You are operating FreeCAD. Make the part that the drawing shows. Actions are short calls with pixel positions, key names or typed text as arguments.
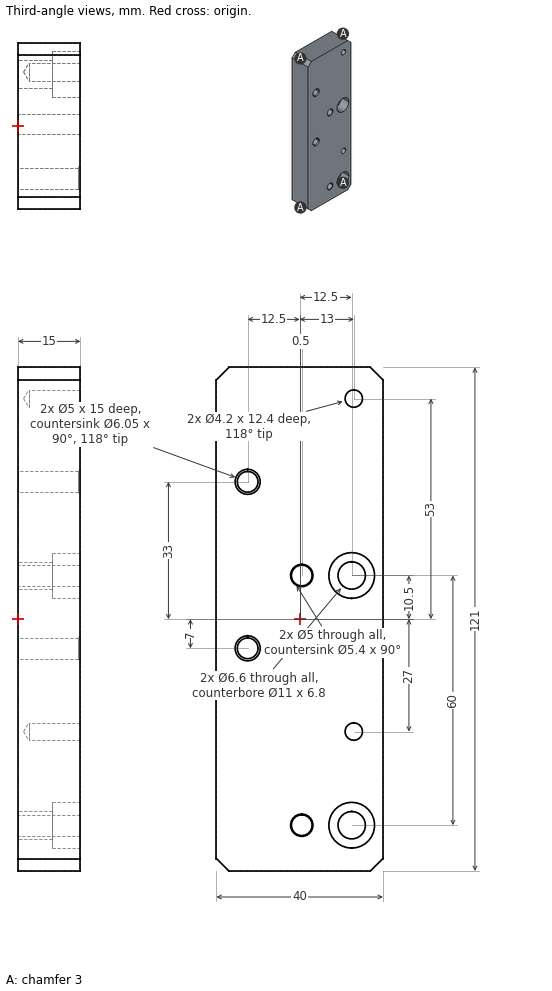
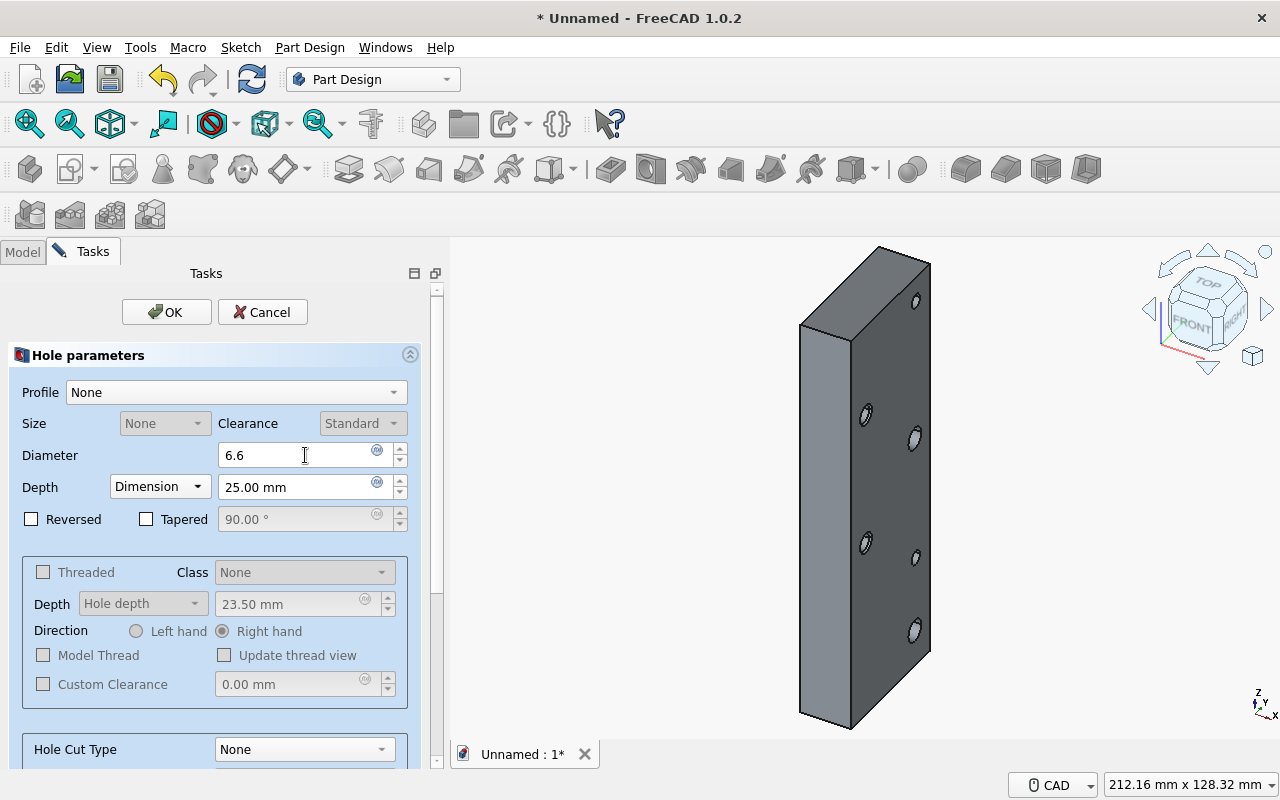
click(161, 486)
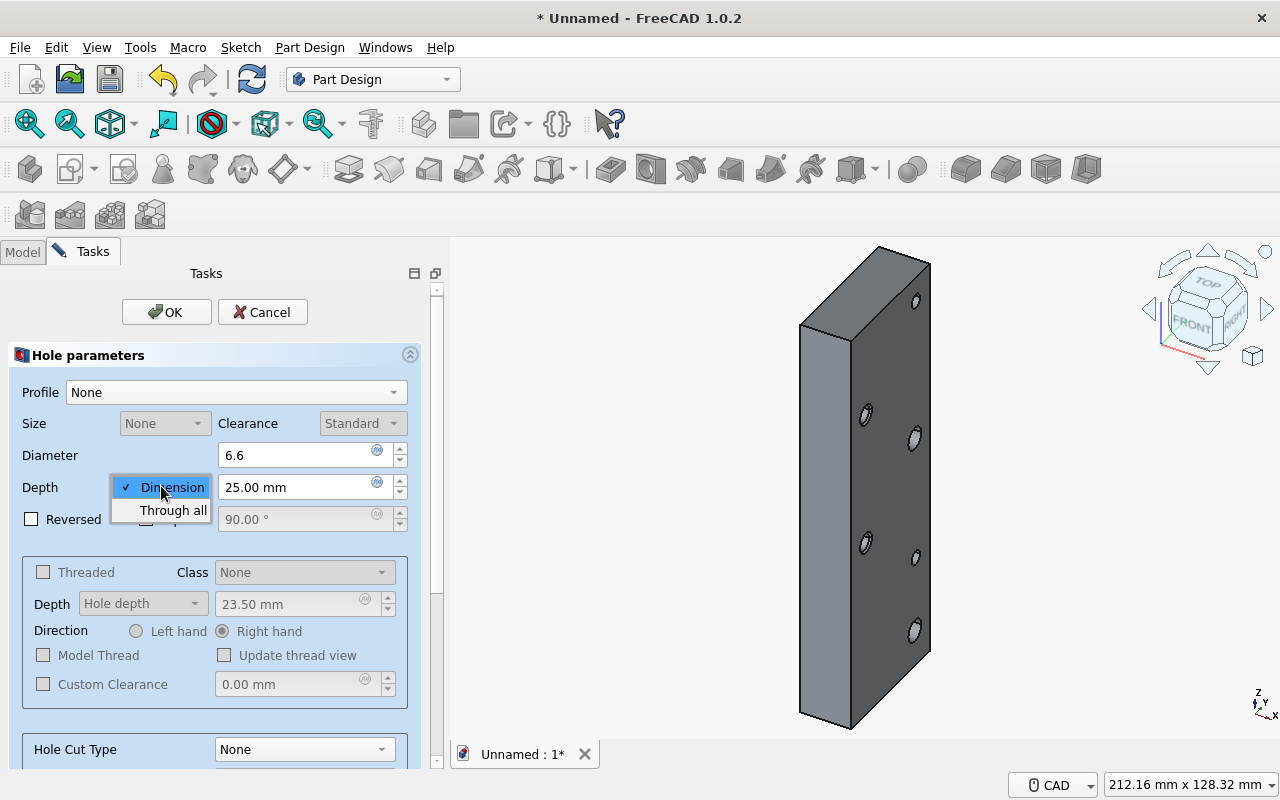
click(160, 510)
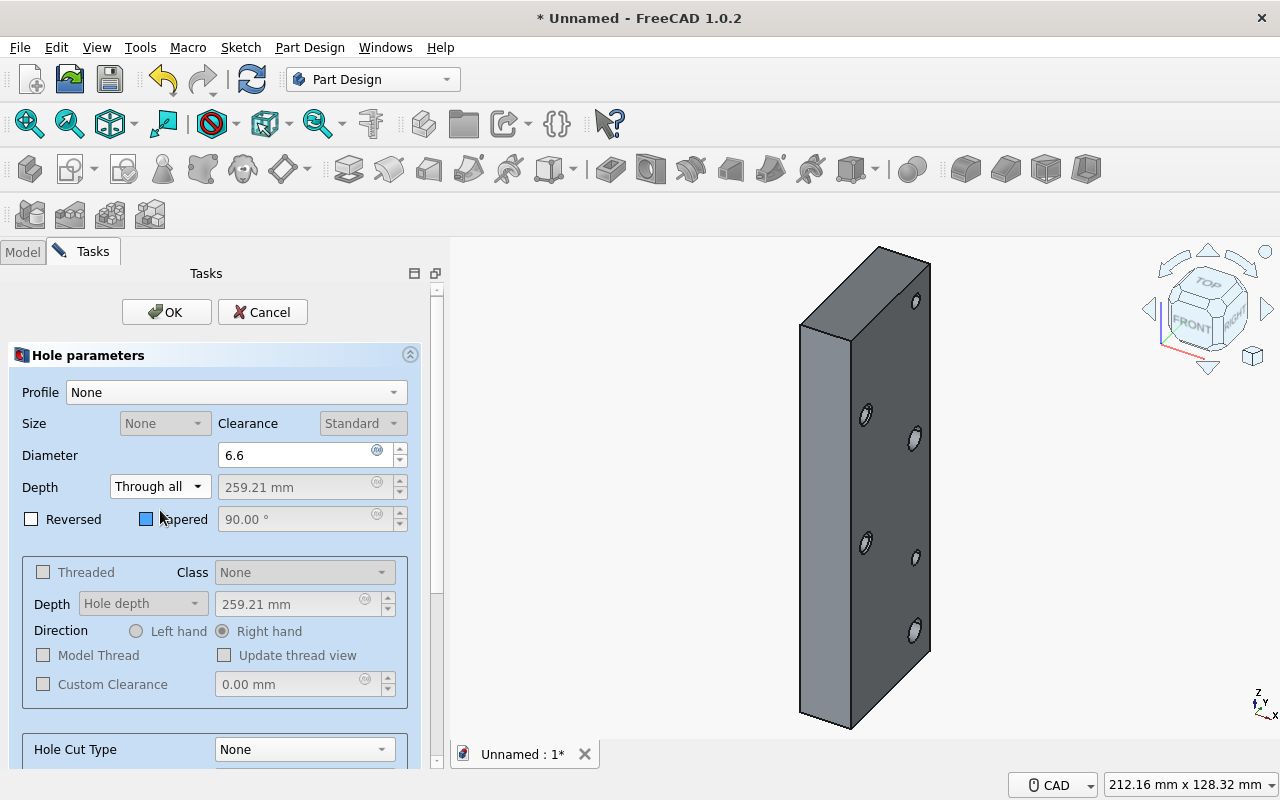
click(306, 750)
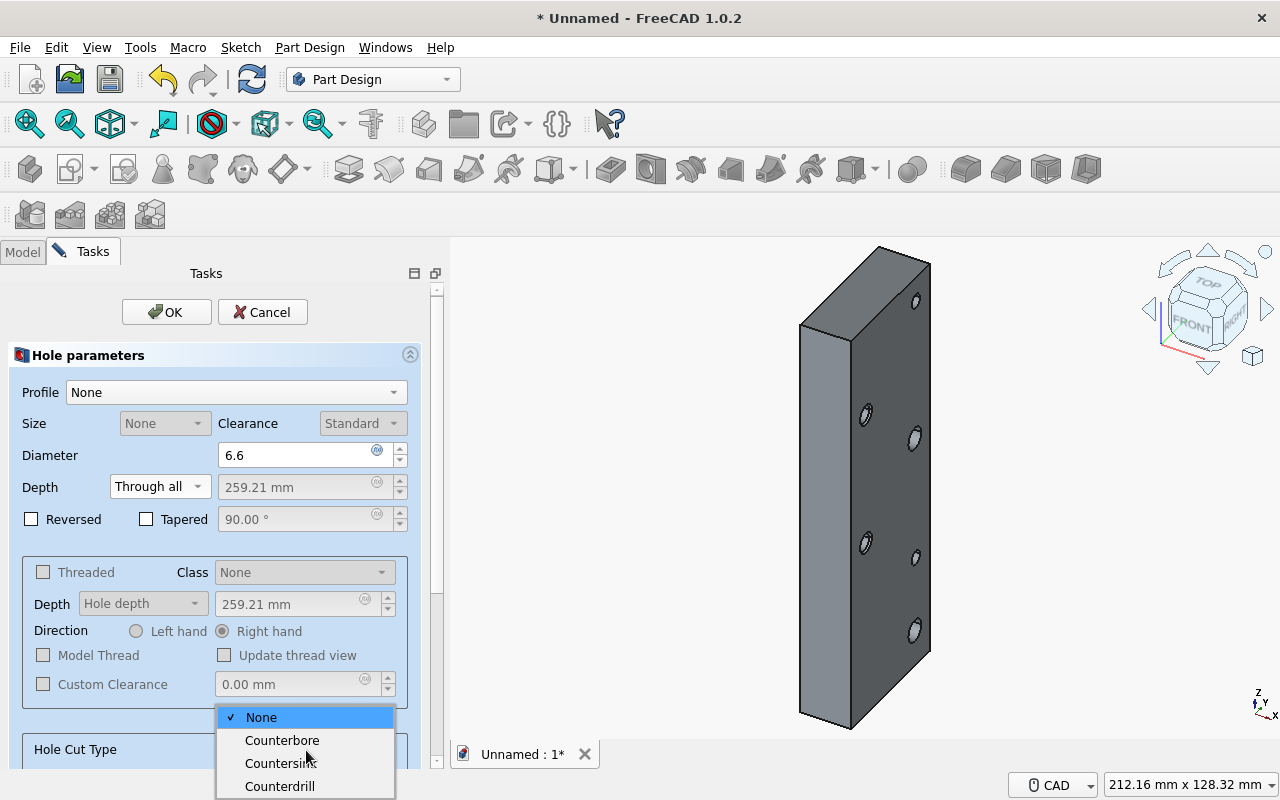
click(304, 740)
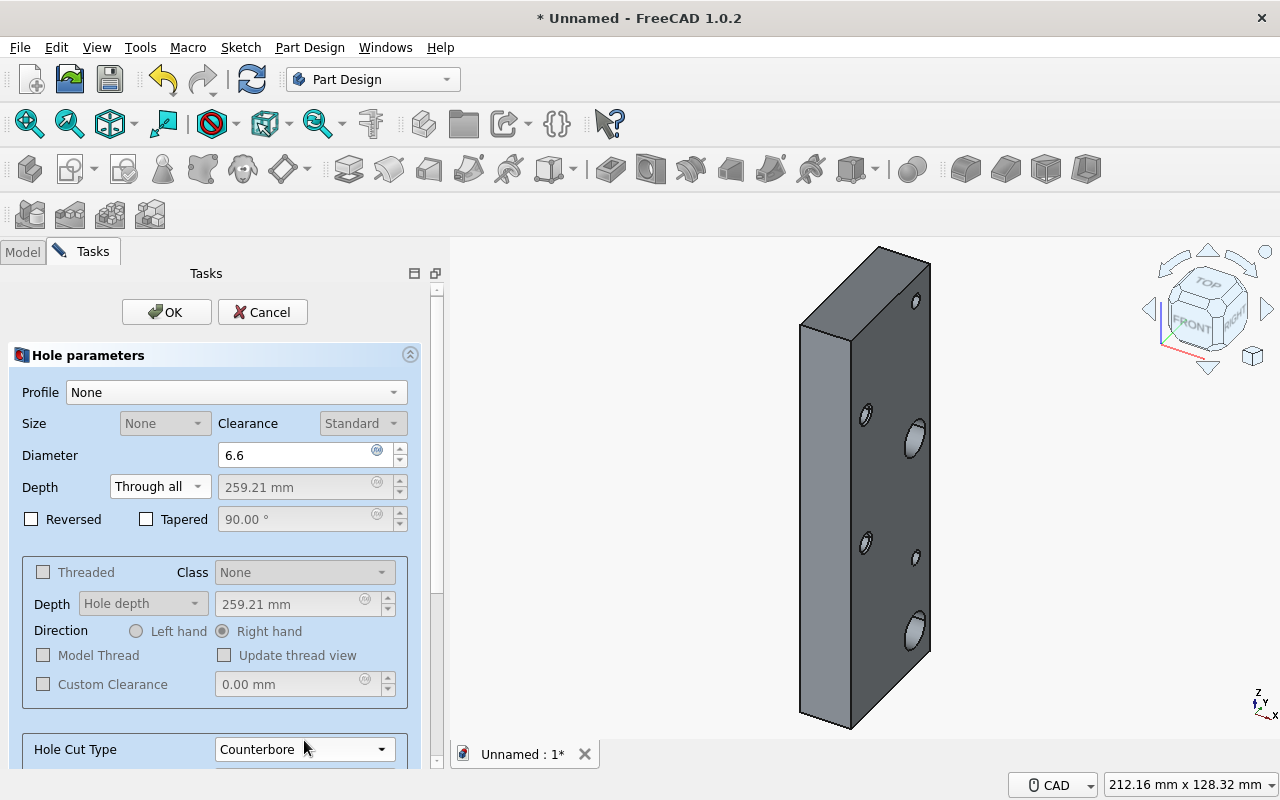
scroll(437, 526, down, 2)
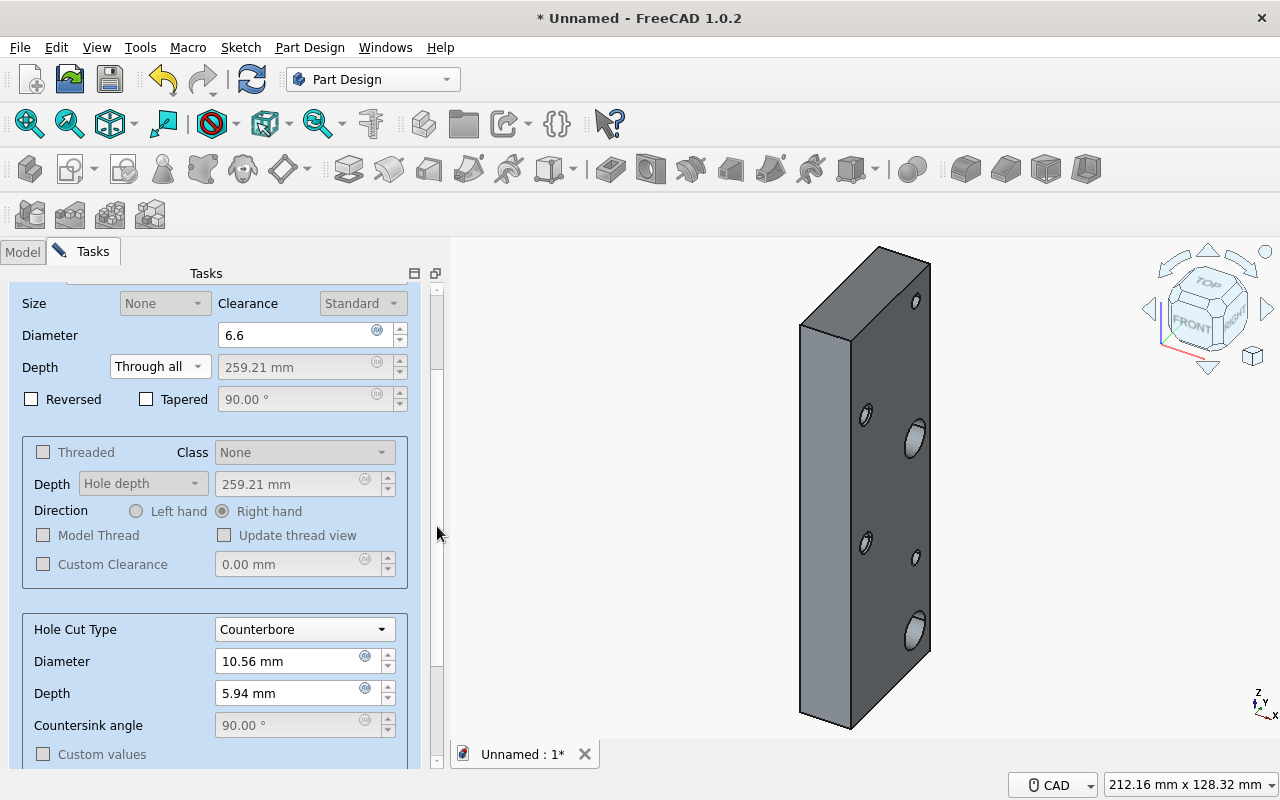
triple_click(298, 661)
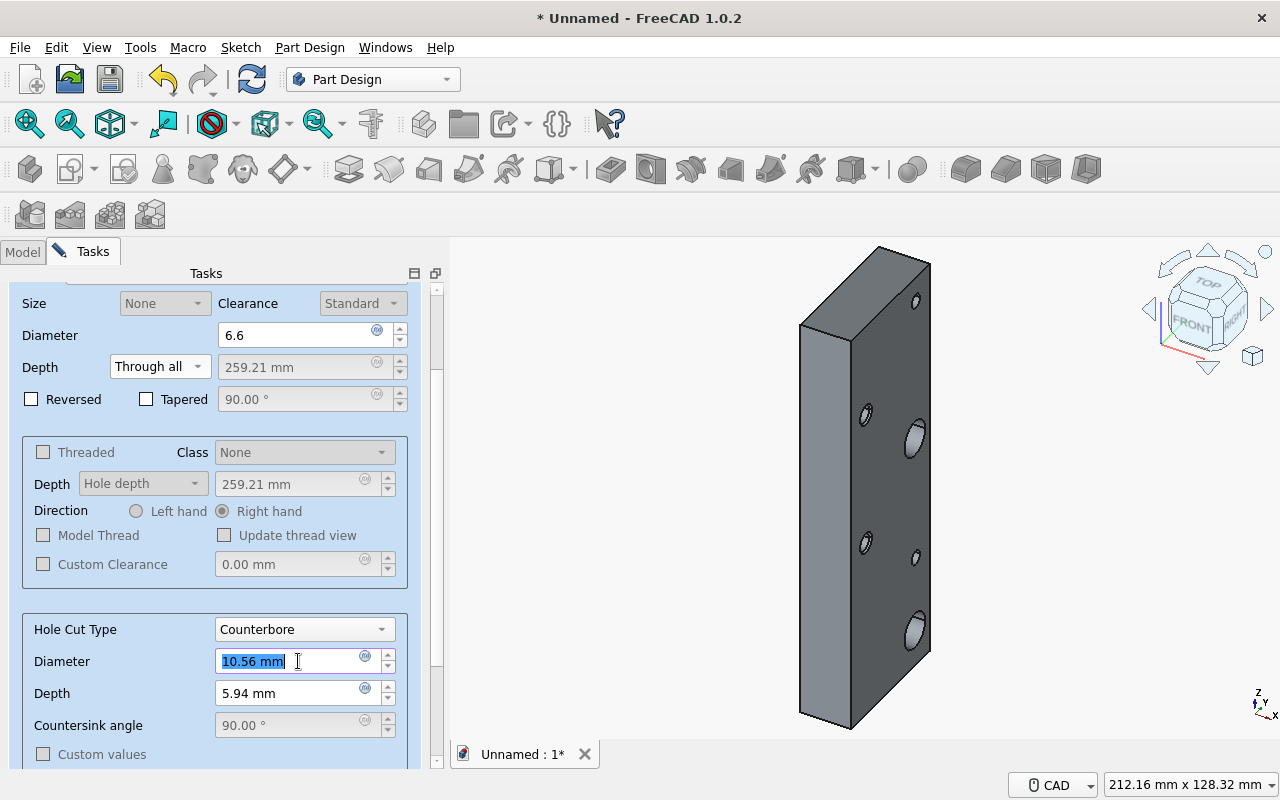
text(11)
key(Tab)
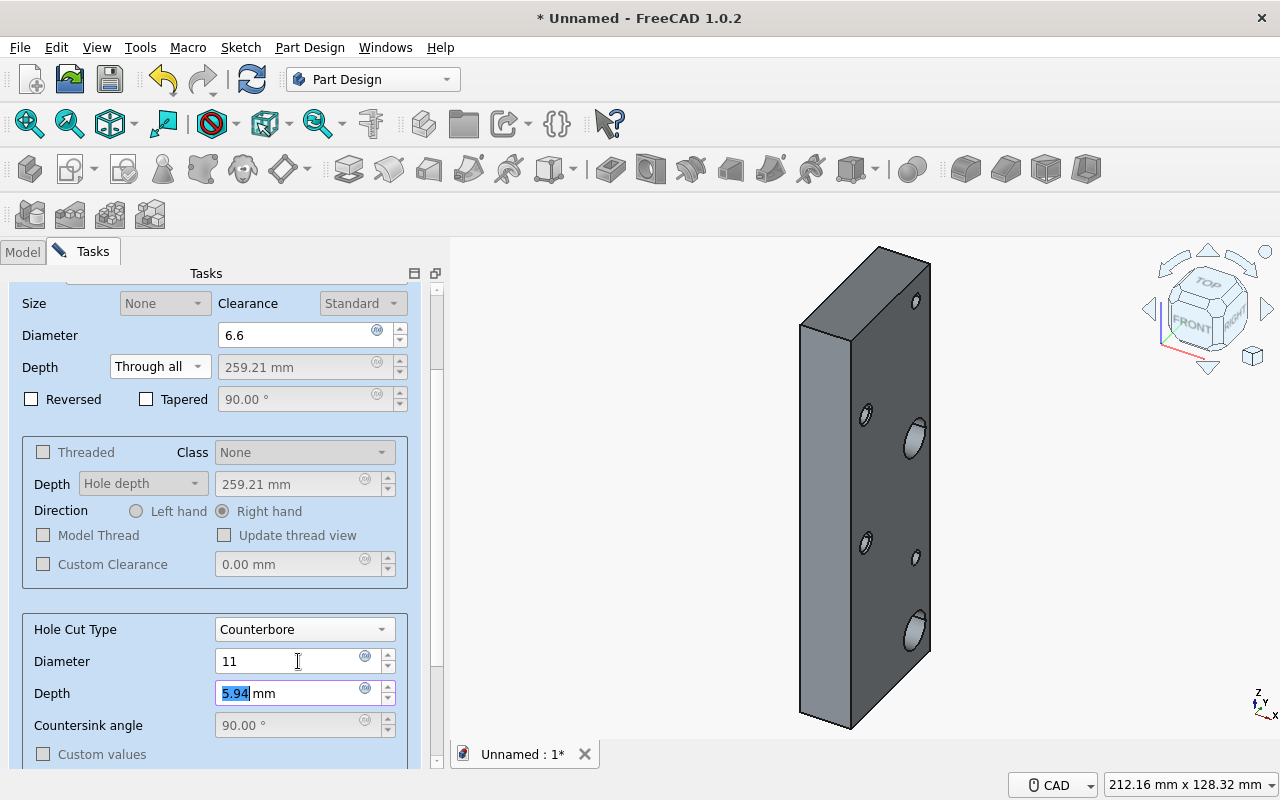
text(6.8)
key(Tab)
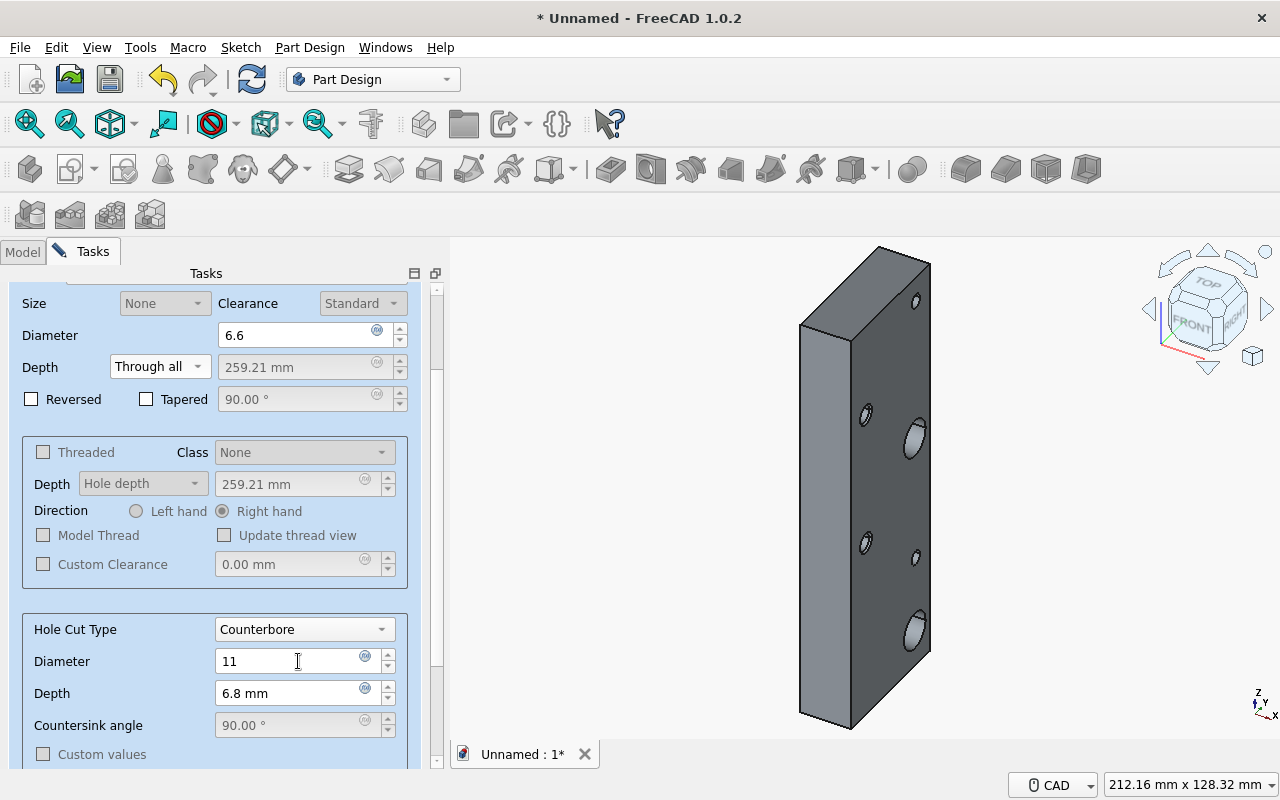
scroll(437, 526, up, 3)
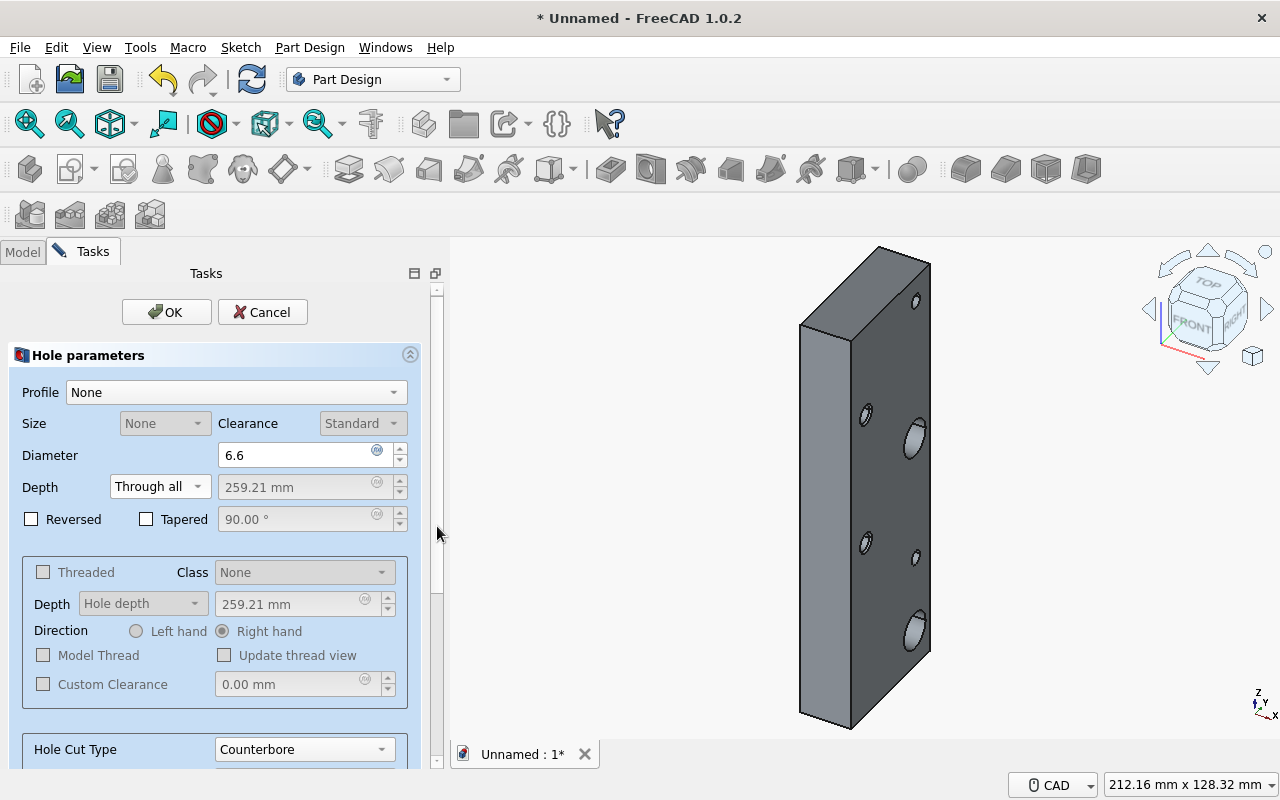
click(167, 312)